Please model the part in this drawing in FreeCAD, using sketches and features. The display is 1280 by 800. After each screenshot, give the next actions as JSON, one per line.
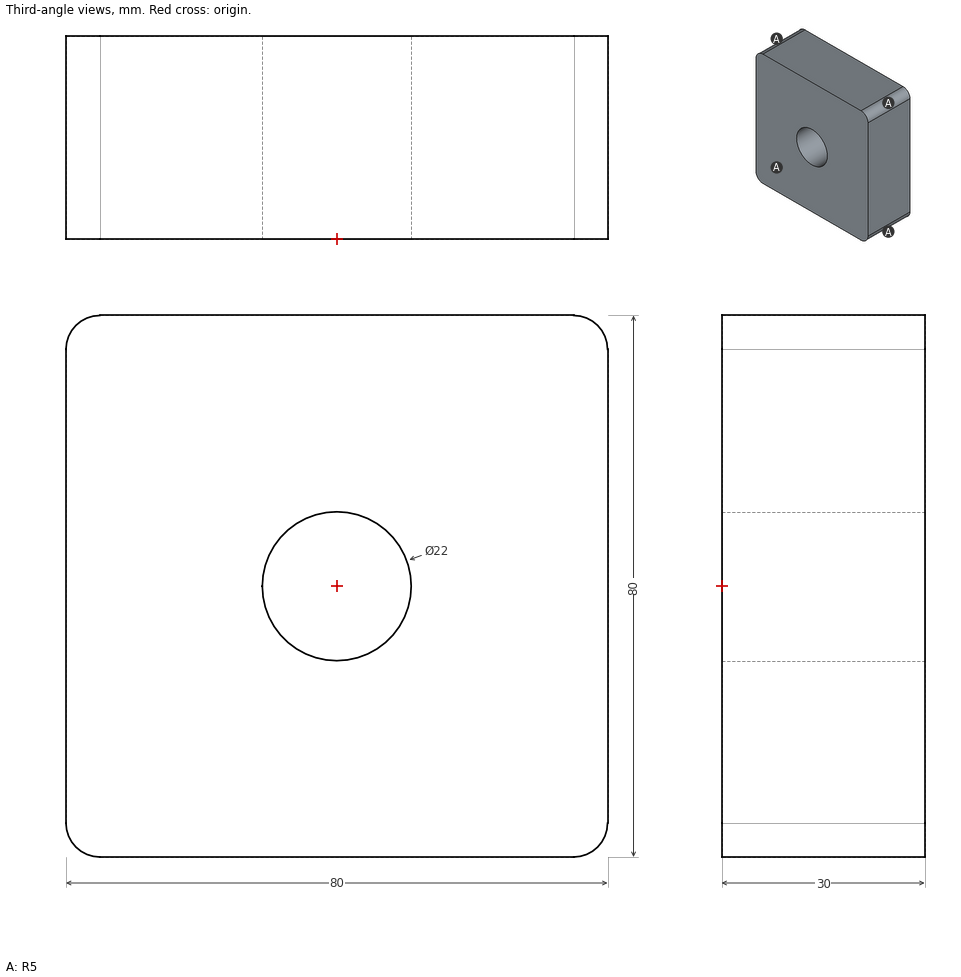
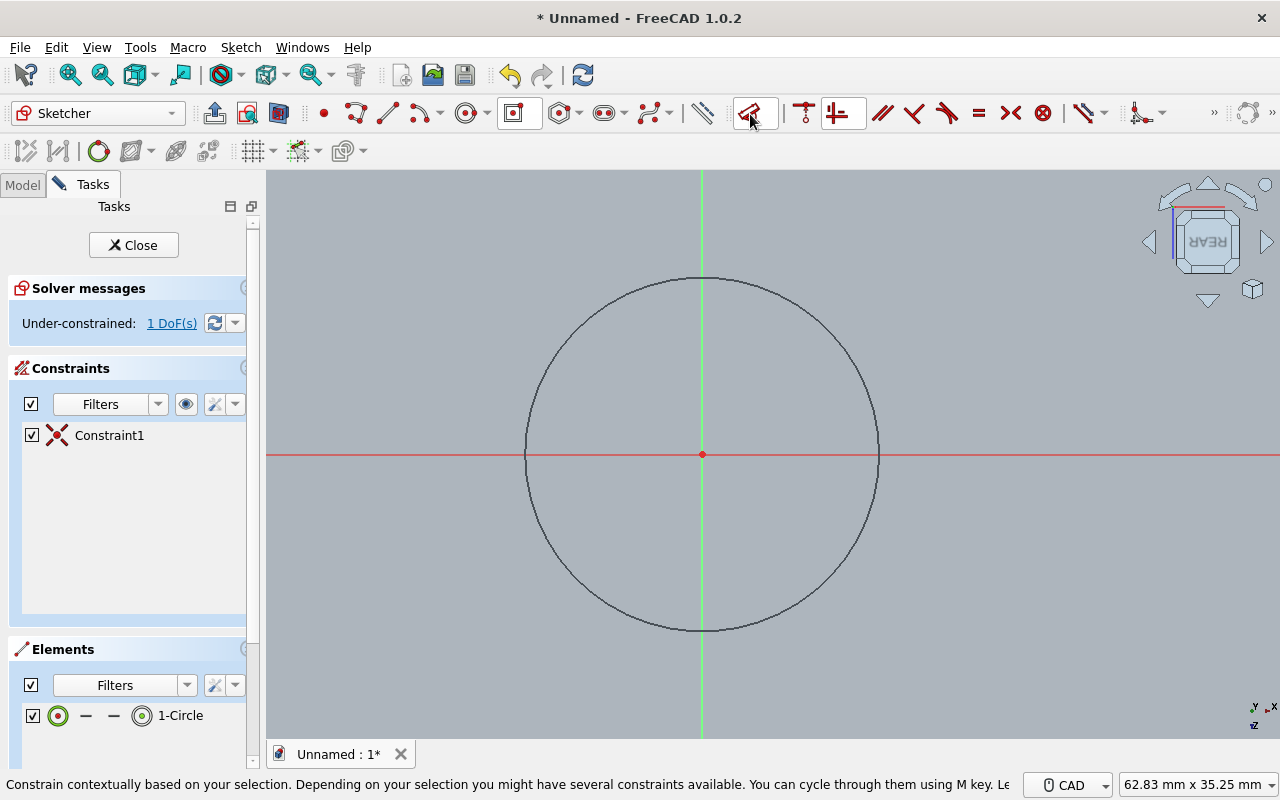
{"action": "left_click", "coordinate": [827, 329]}
{"action": "left_click", "coordinate": [850, 306]}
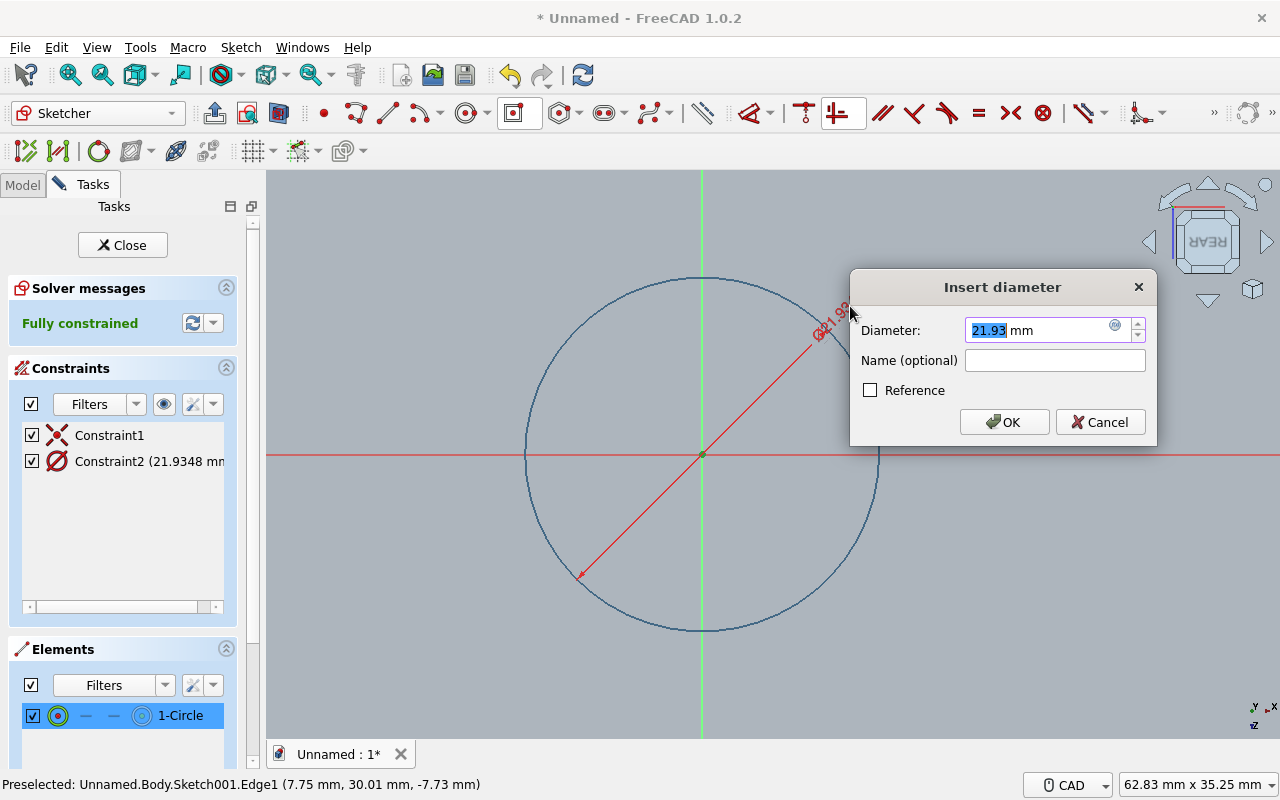
{"action": "type", "text": "22"}
{"action": "key", "text": "Return"}
{"action": "key", "text": "Escape"}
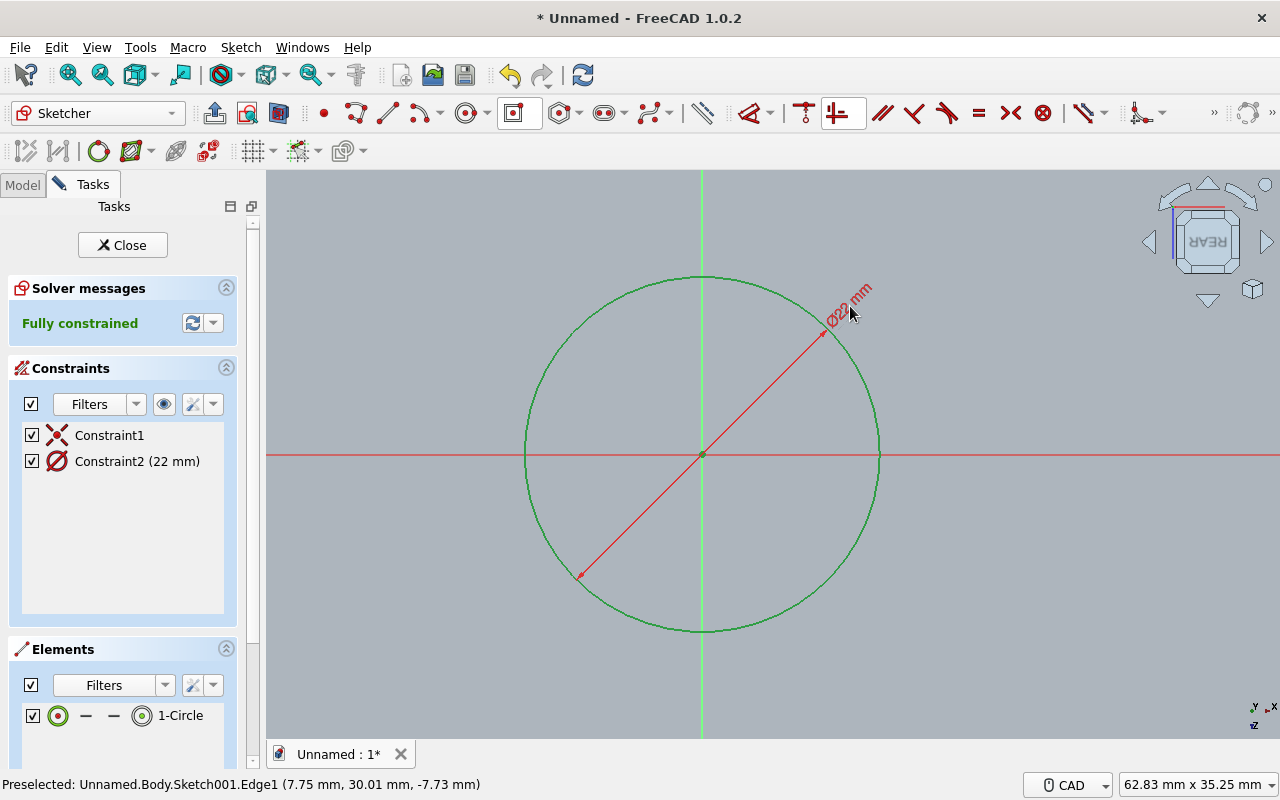
{"action": "left_click", "coordinate": [123, 245]}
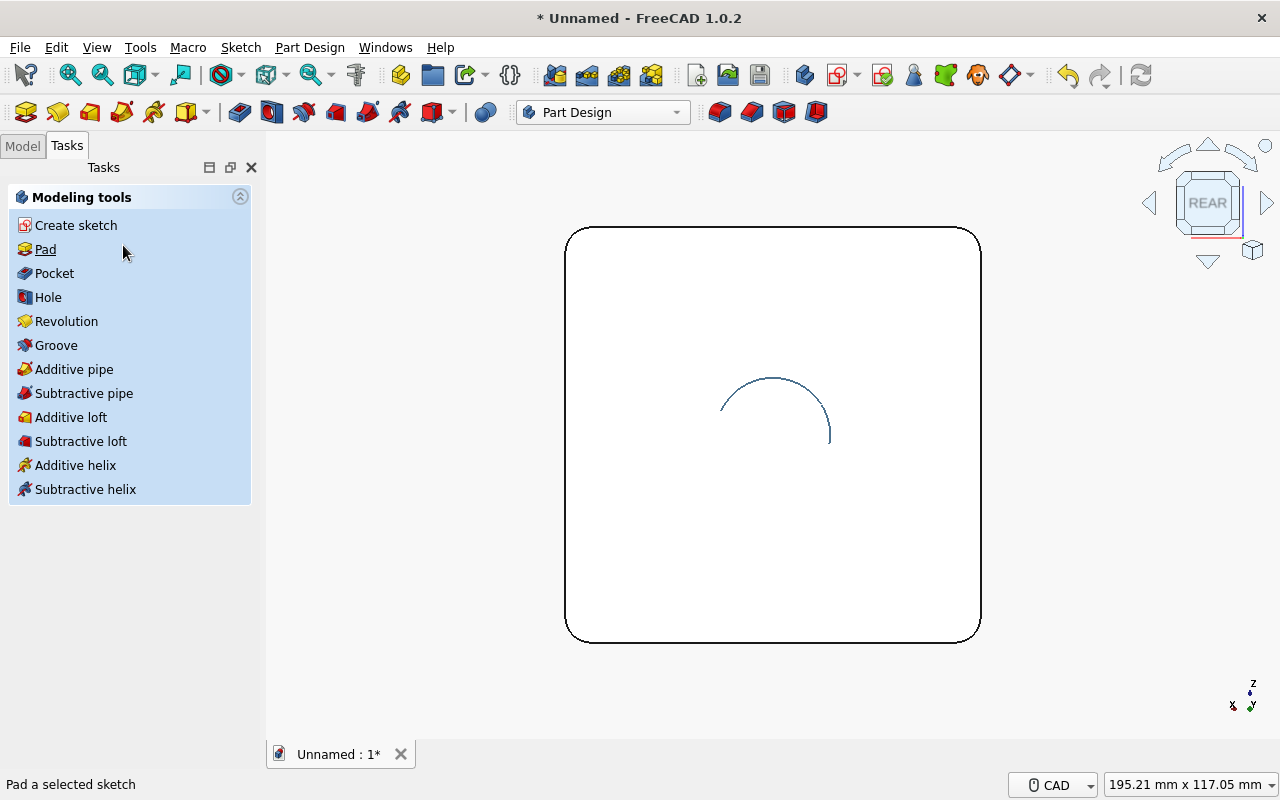
{"action": "left_click", "coordinate": [240, 112]}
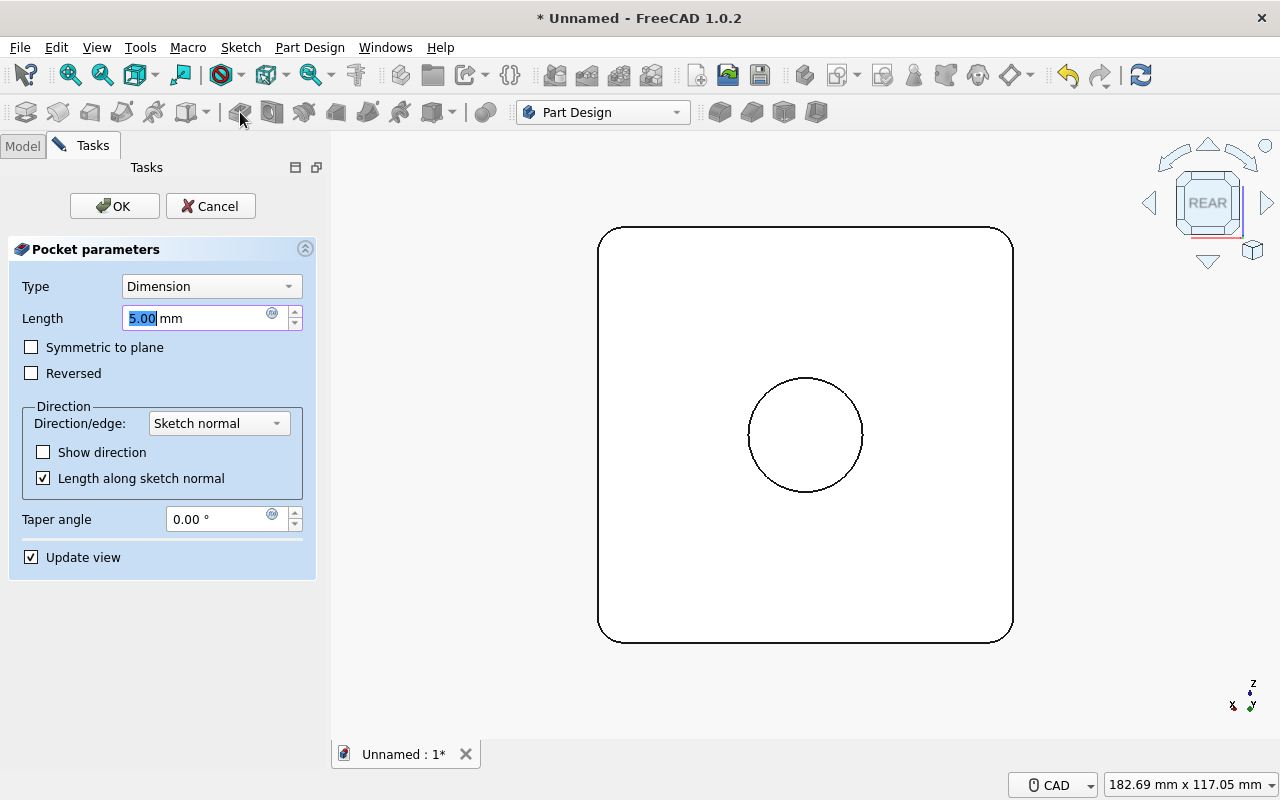
{"action": "left_click", "coordinate": [212, 286]}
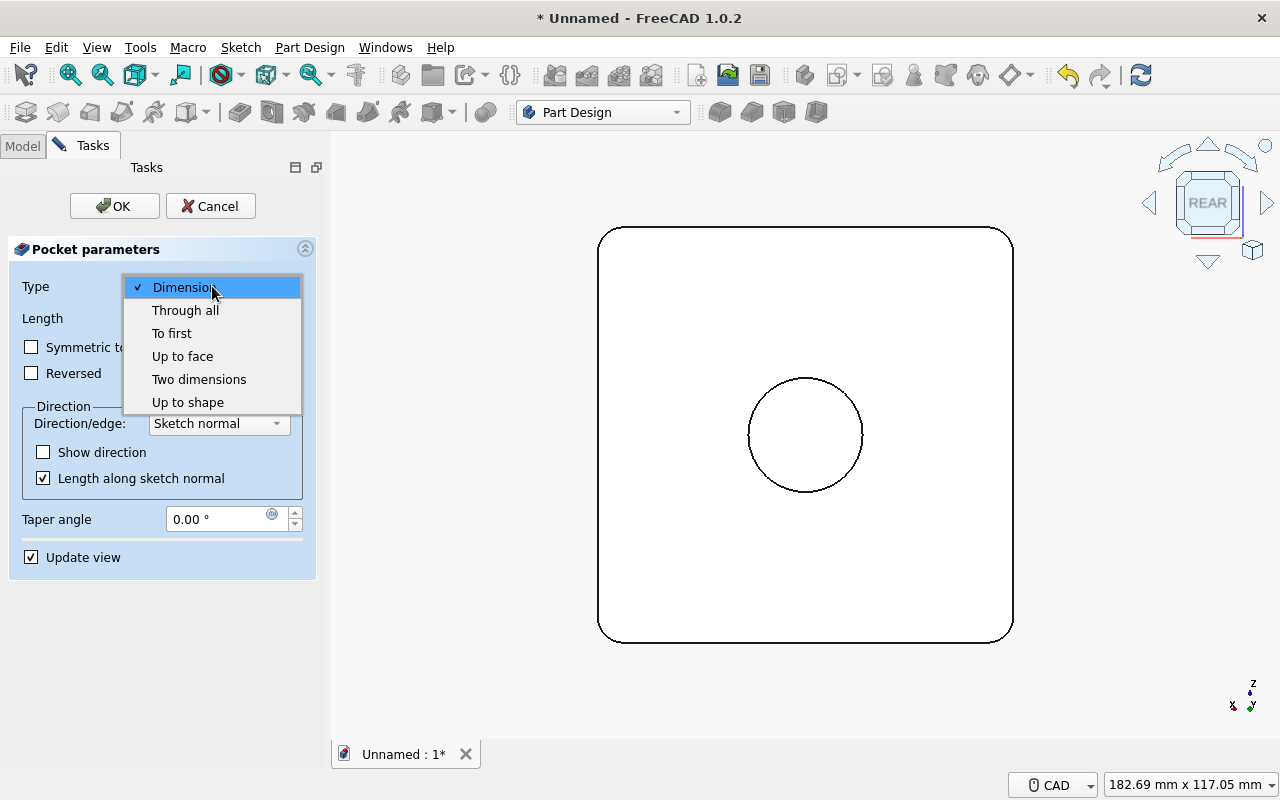
{"action": "left_click", "coordinate": [212, 310]}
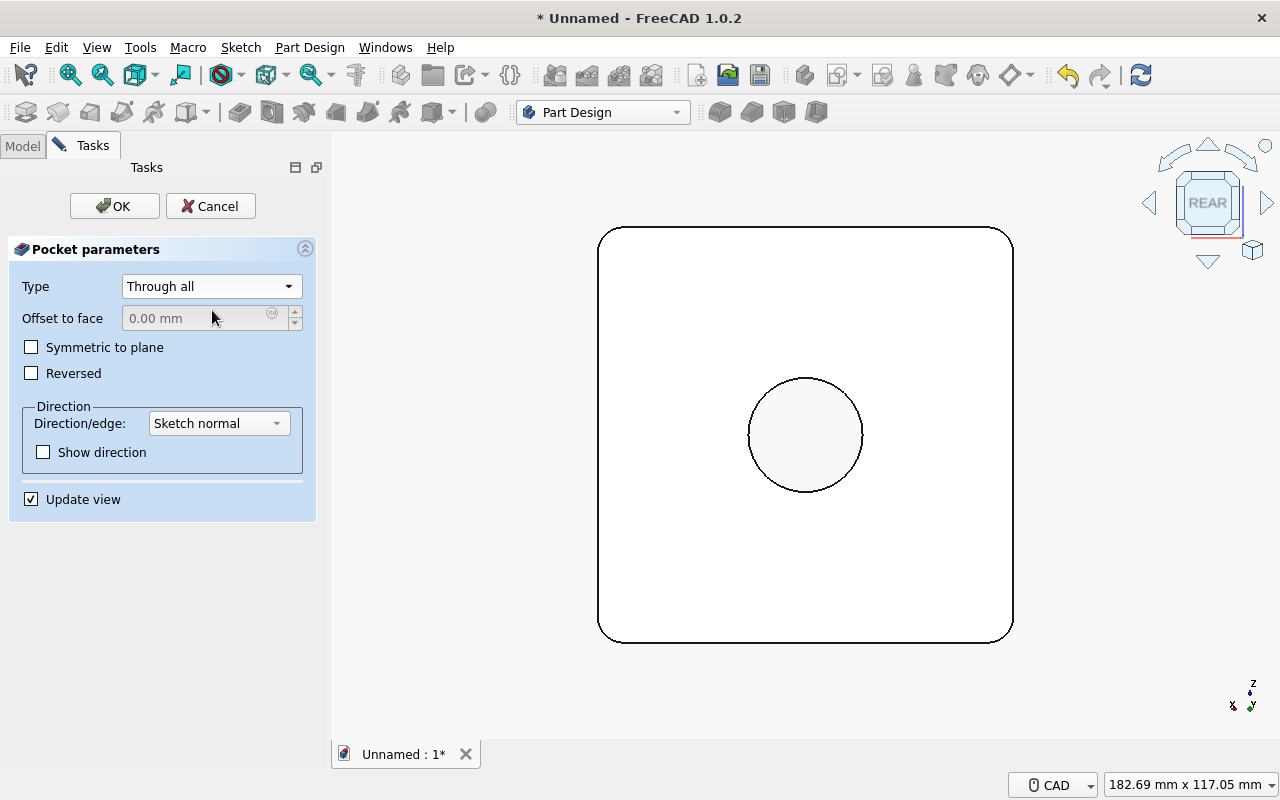
{"action": "left_click", "coordinate": [115, 206]}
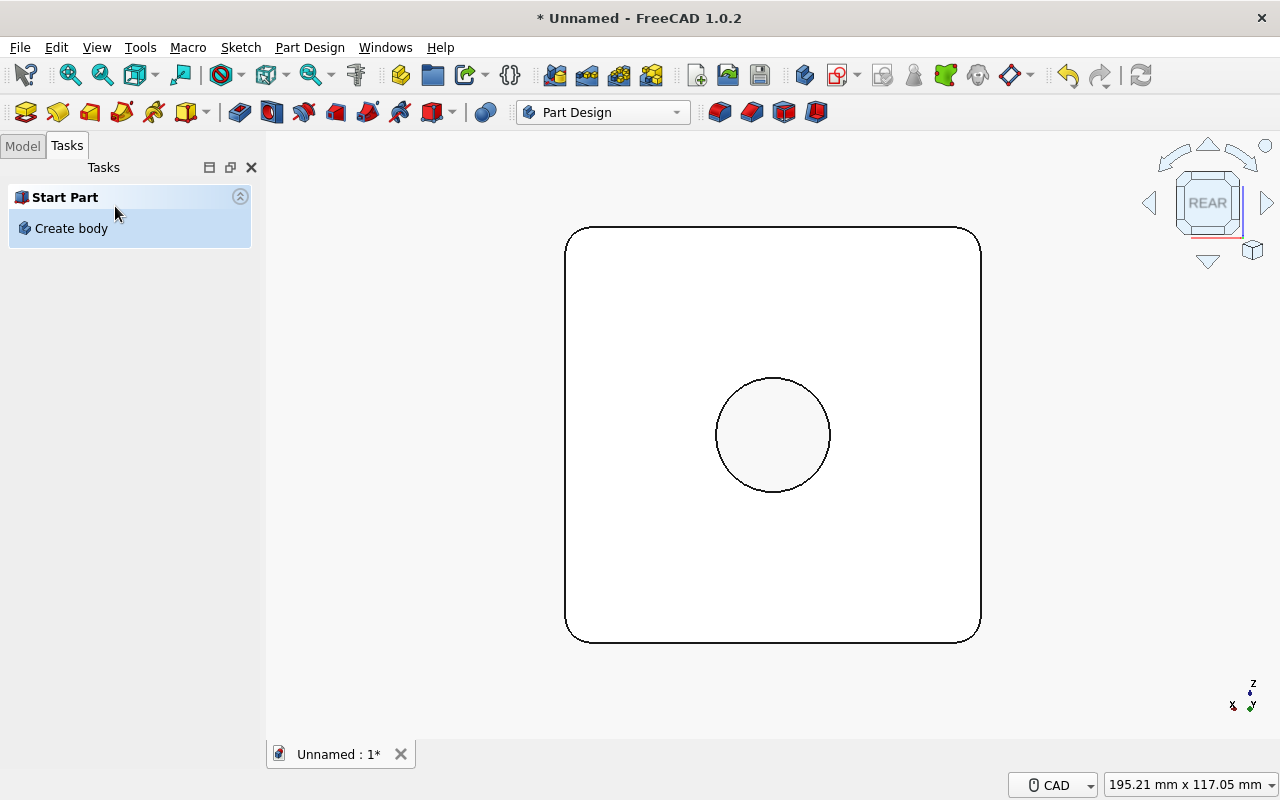
{"action": "key", "text": "0"}